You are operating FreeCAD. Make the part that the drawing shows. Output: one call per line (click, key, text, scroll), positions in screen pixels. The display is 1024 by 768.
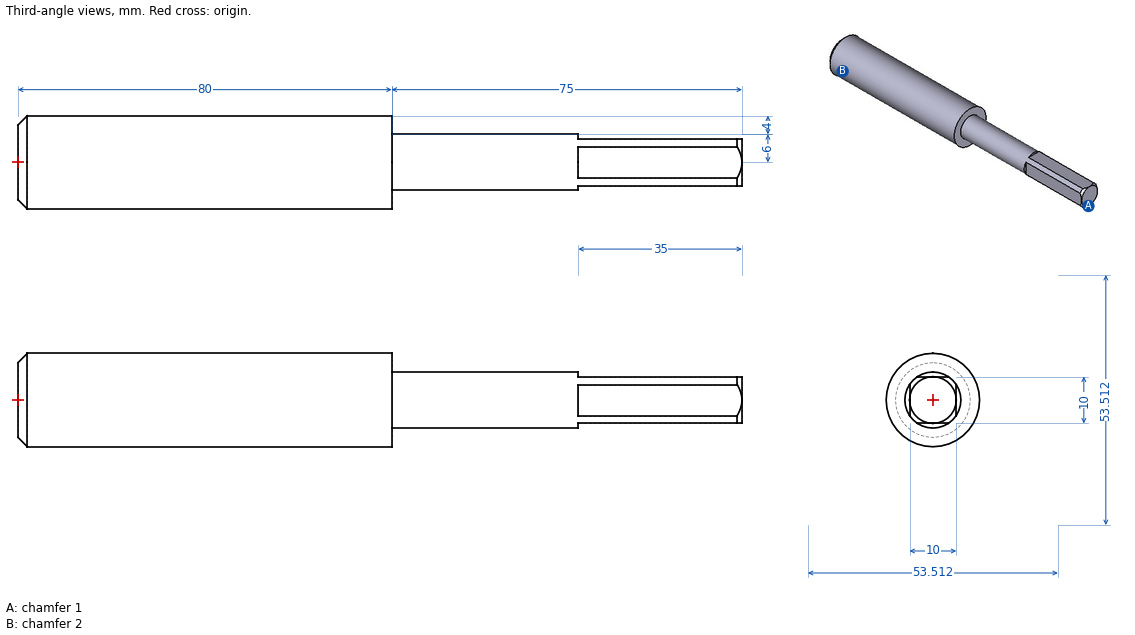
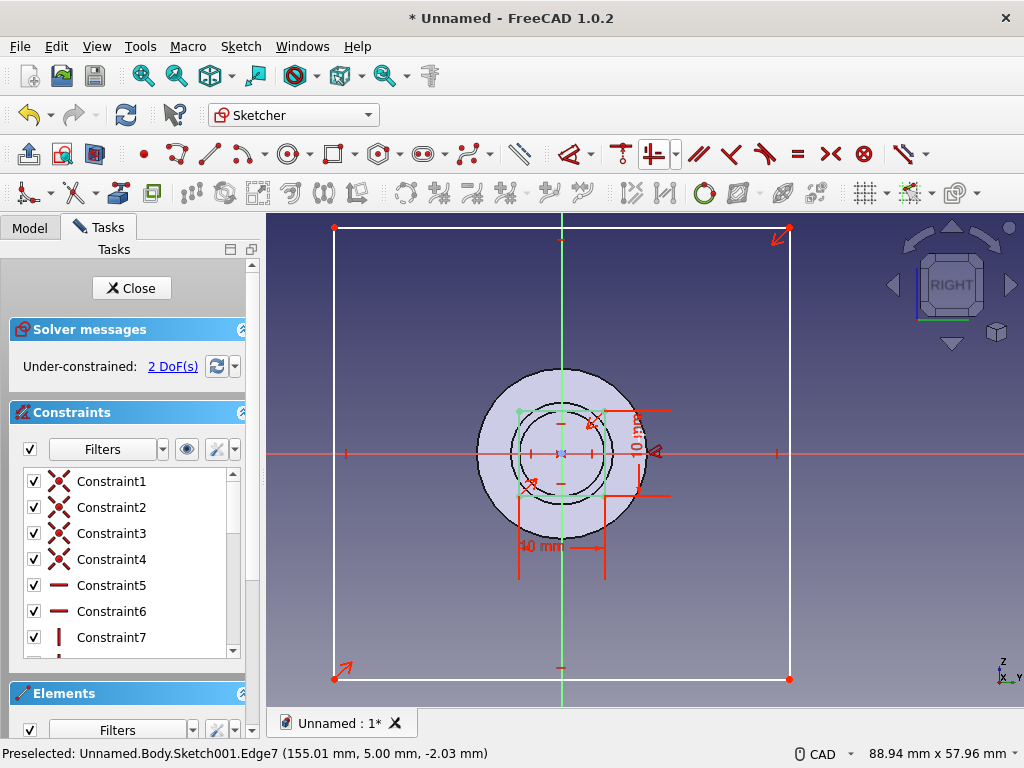
scroll(606, 473, down, 2)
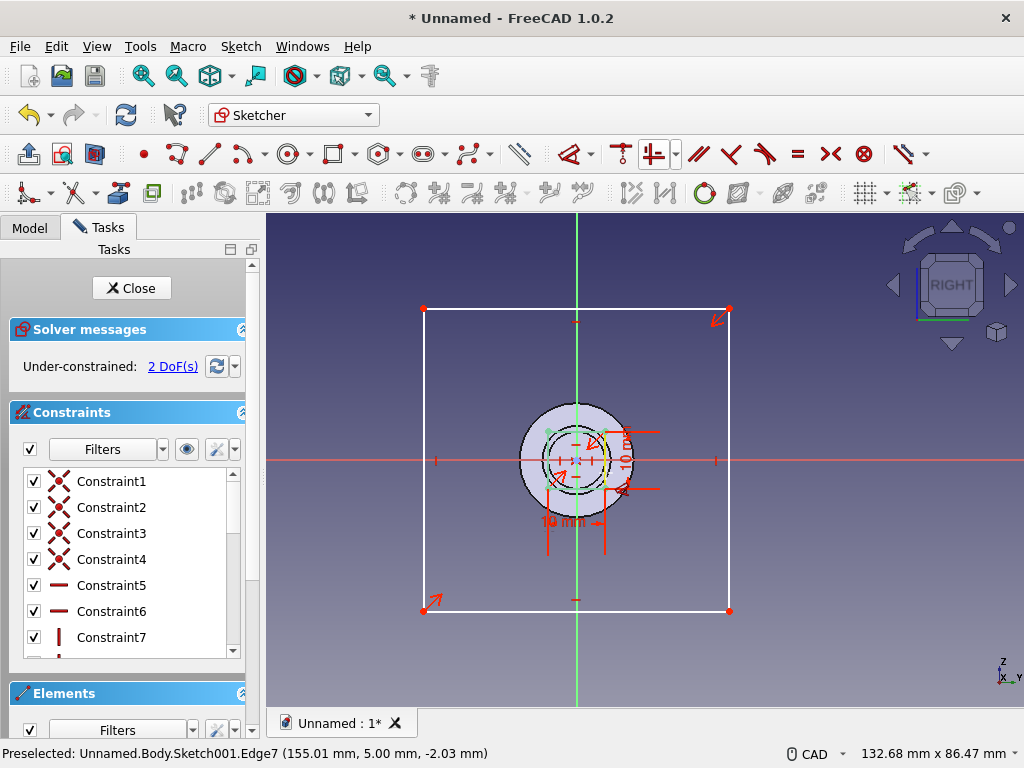
click(515, 612)
click(506, 646)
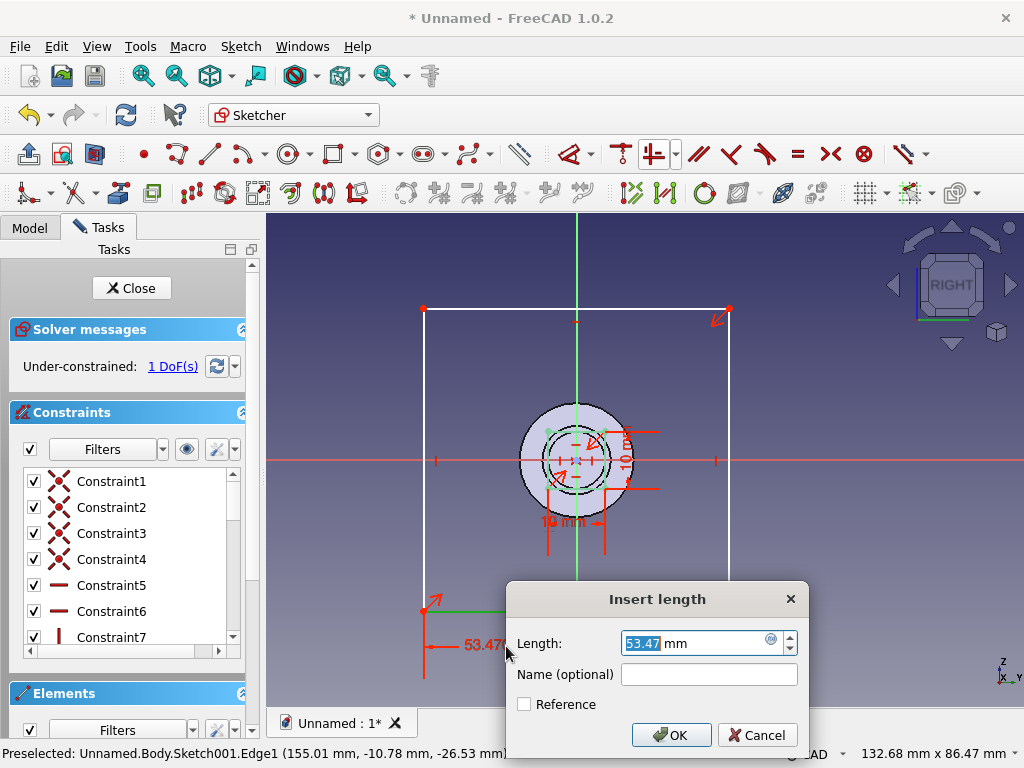
text(53.512)
key(Return)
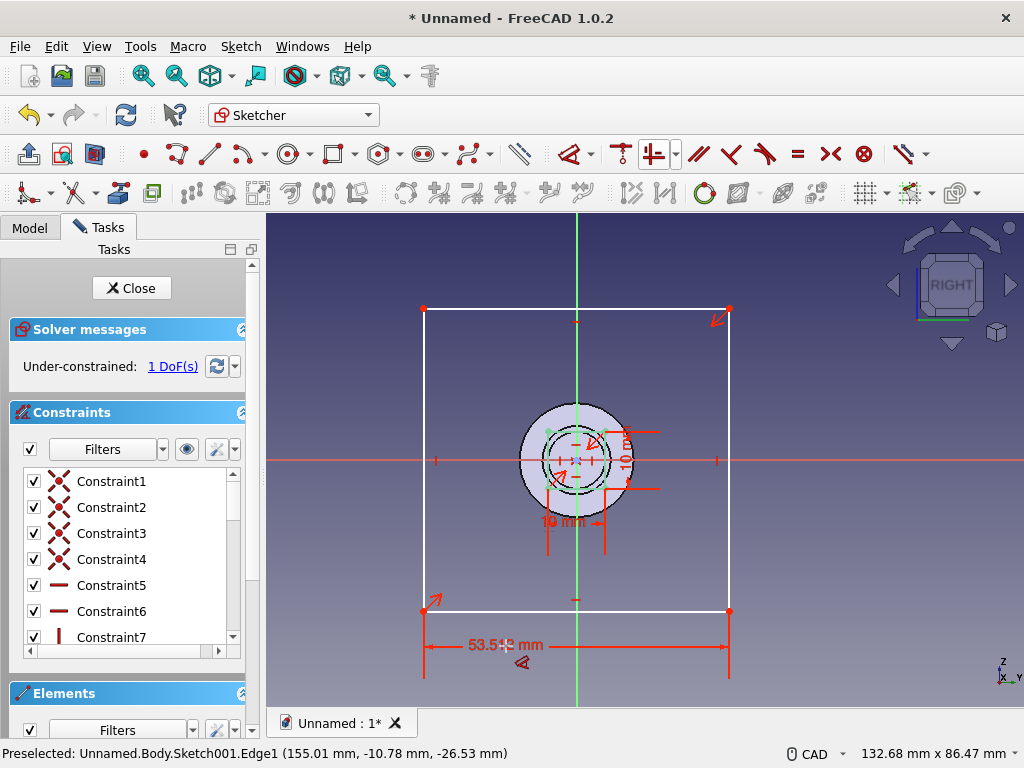
click(729, 521)
click(763, 391)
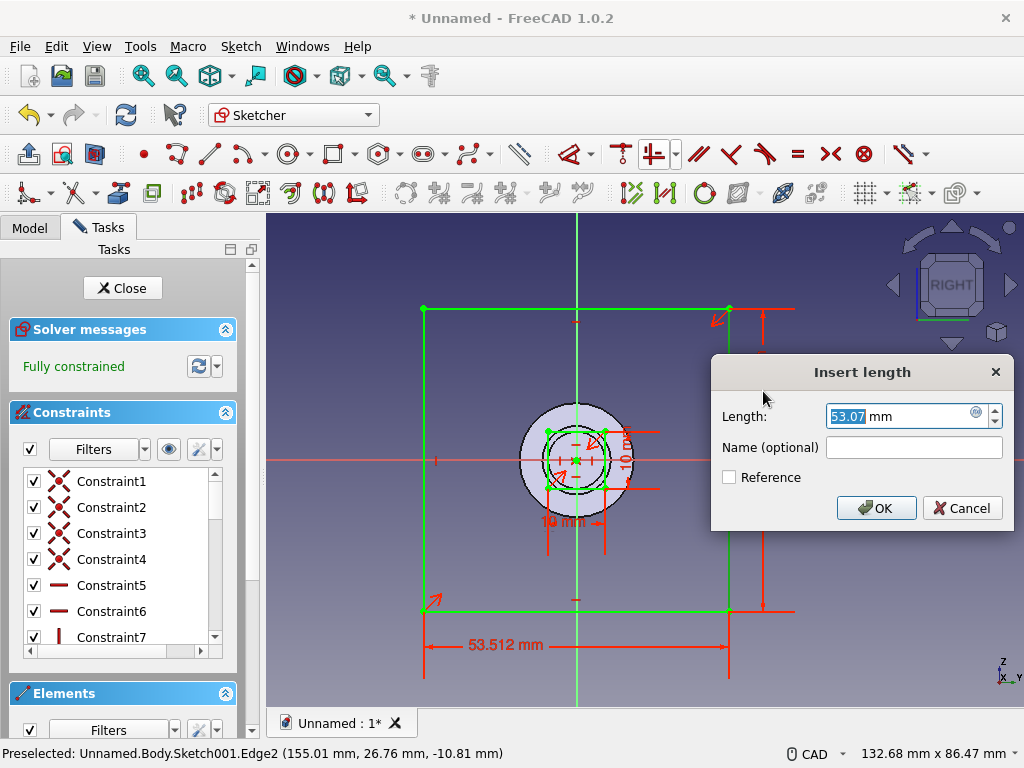
text(53.512)
key(Return)
key(Escape)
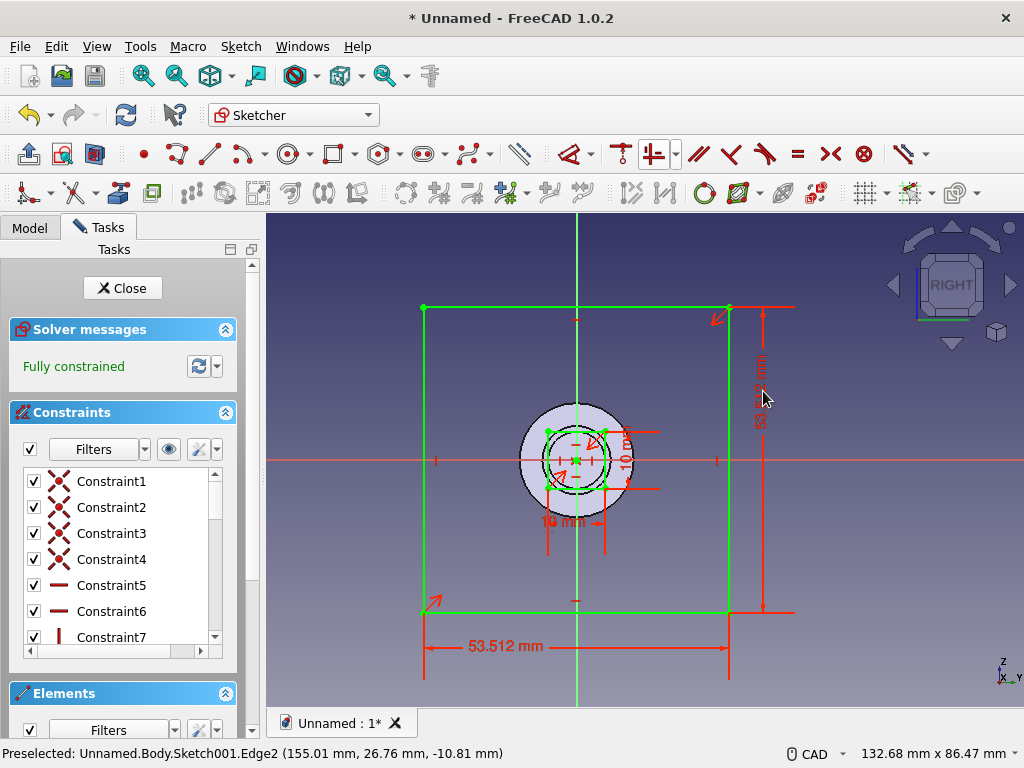
click(123, 288)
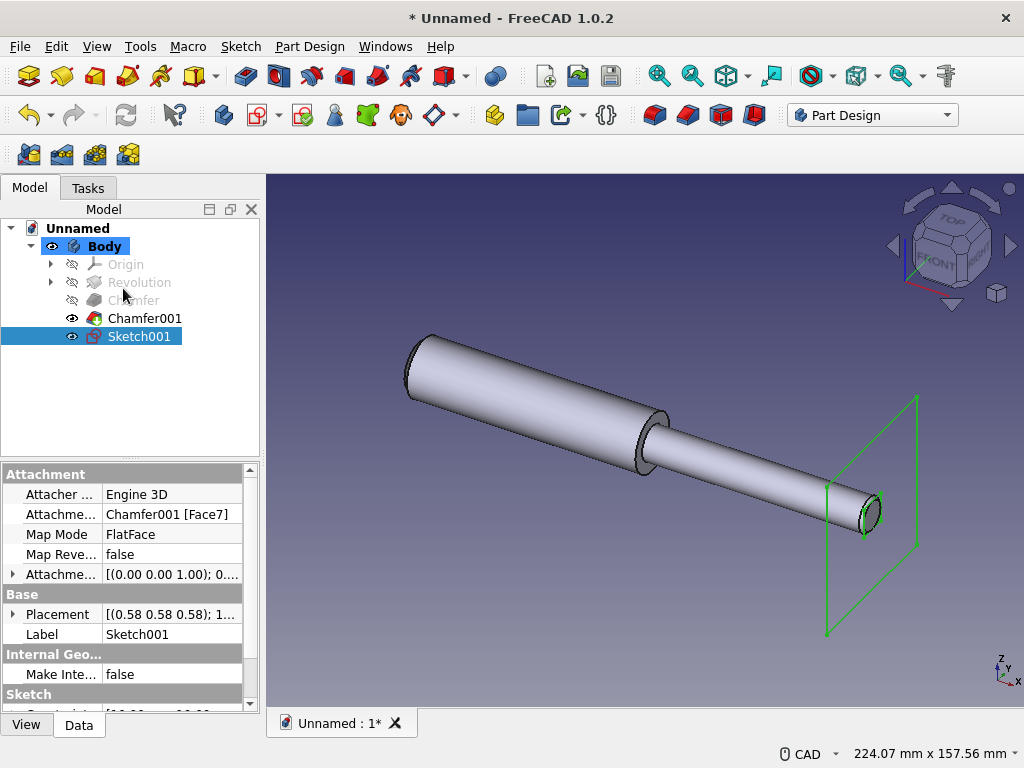
click(246, 76)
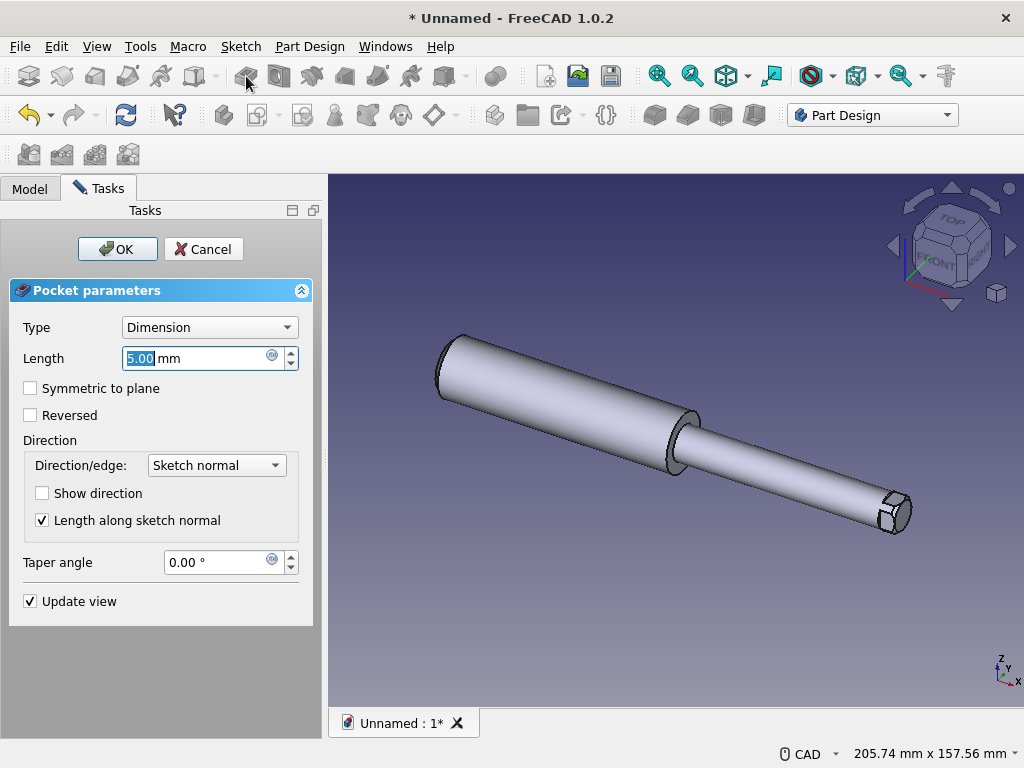
text(35)
key(Tab)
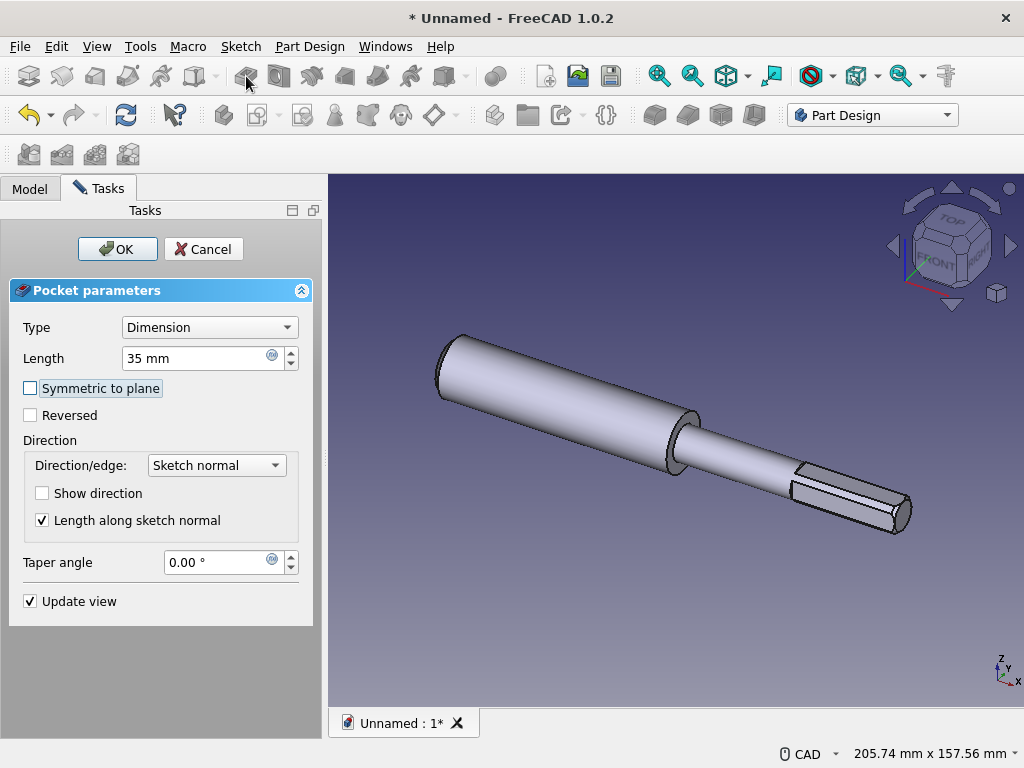
click(118, 249)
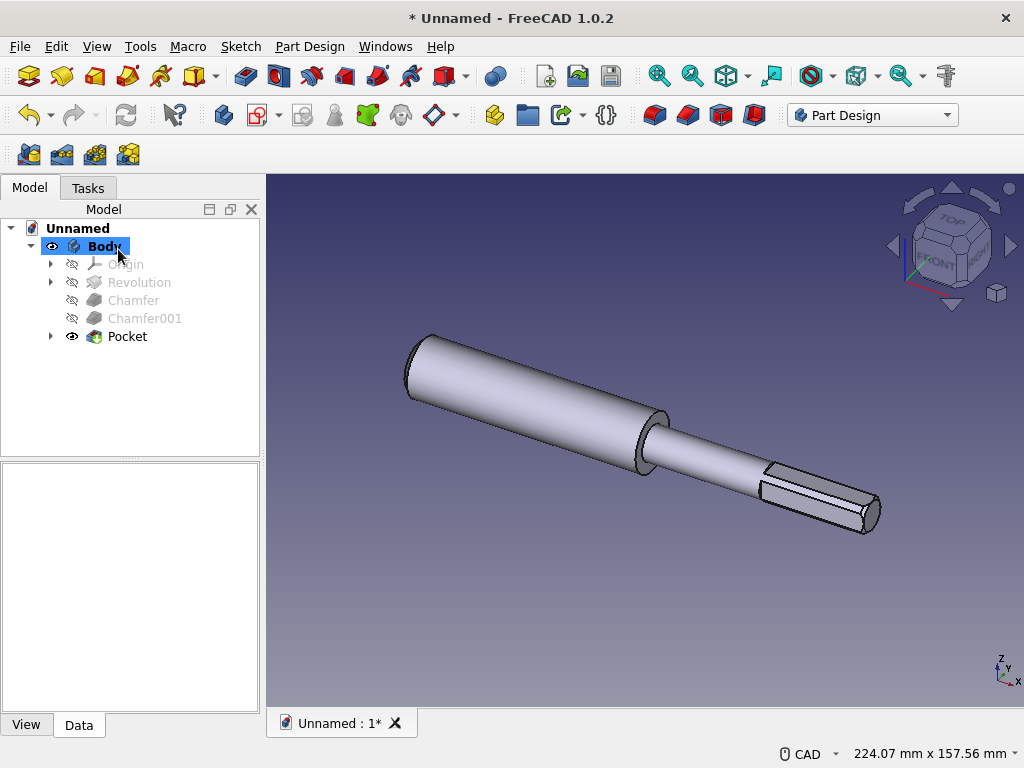
key(0)